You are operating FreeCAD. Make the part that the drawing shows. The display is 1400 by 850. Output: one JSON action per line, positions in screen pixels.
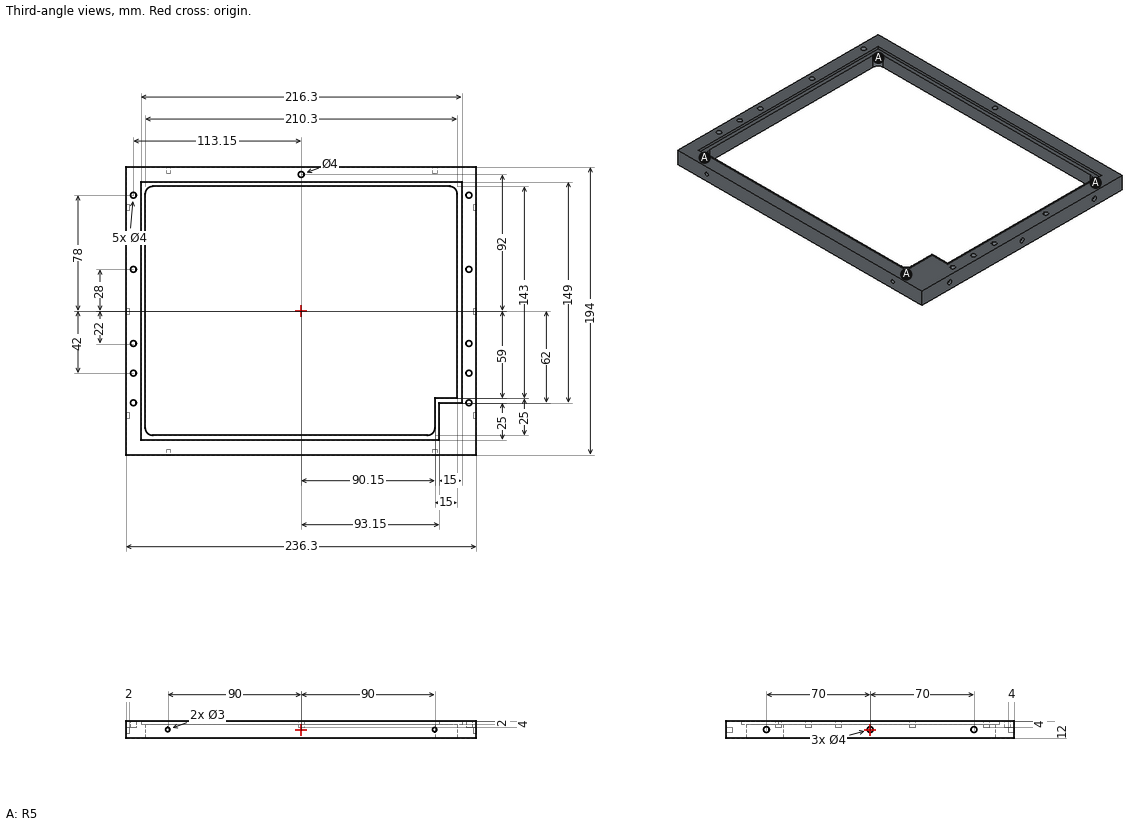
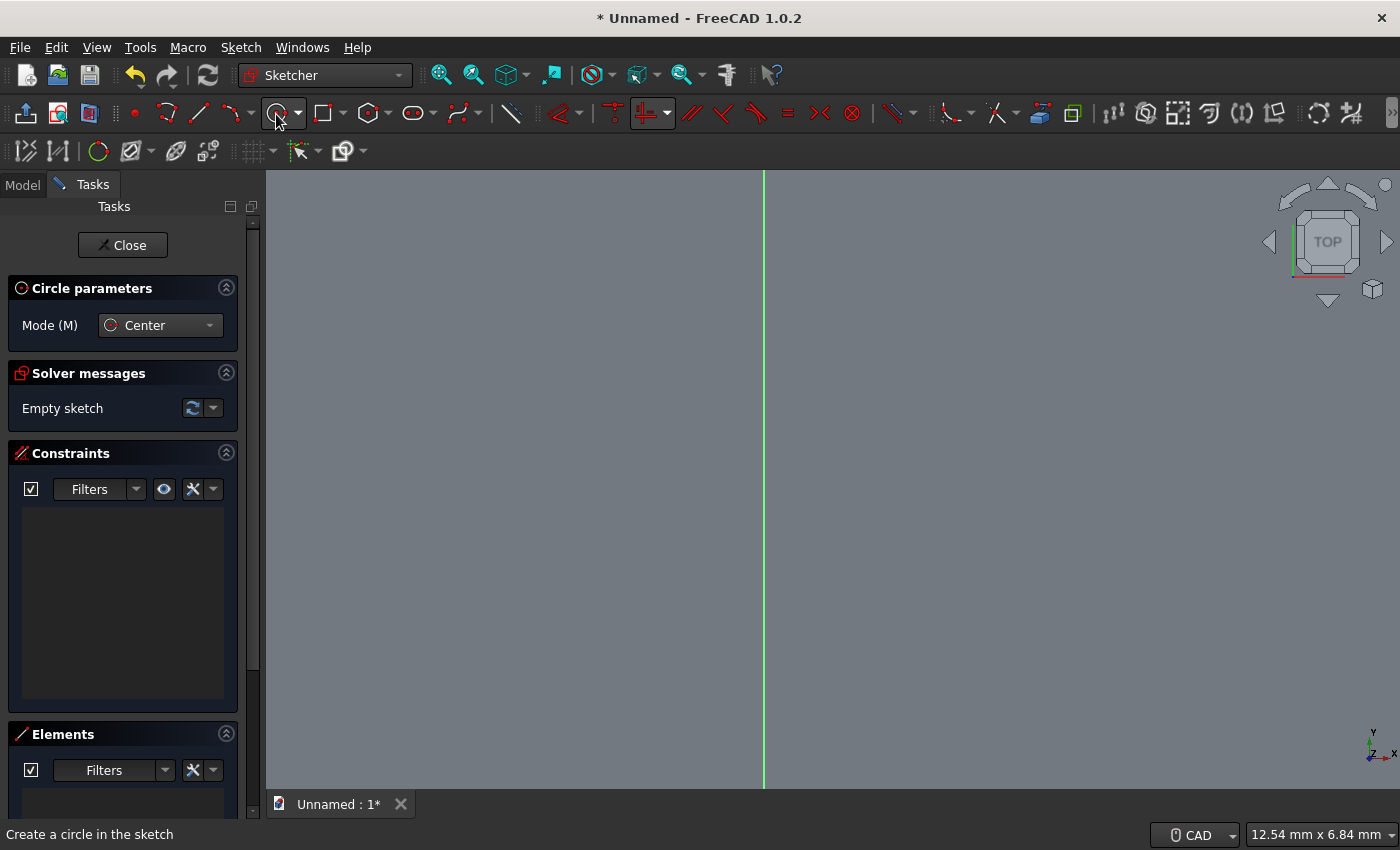
{"action": "left_click", "coordinate": [764, 479]}
{"action": "left_click", "coordinate": [892, 351]}
{"action": "key", "text": "Escape"}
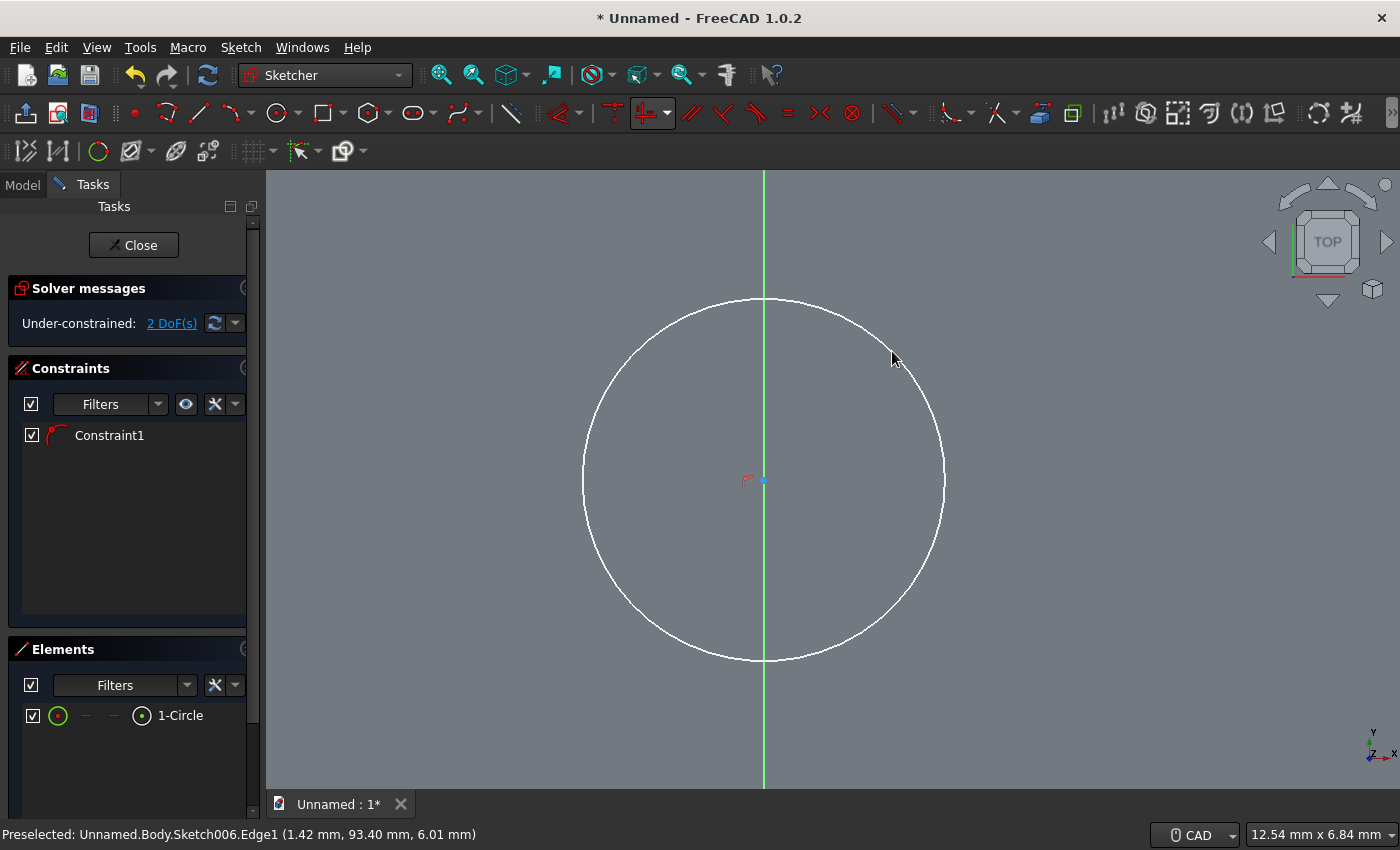
{"action": "left_click", "coordinate": [558, 114]}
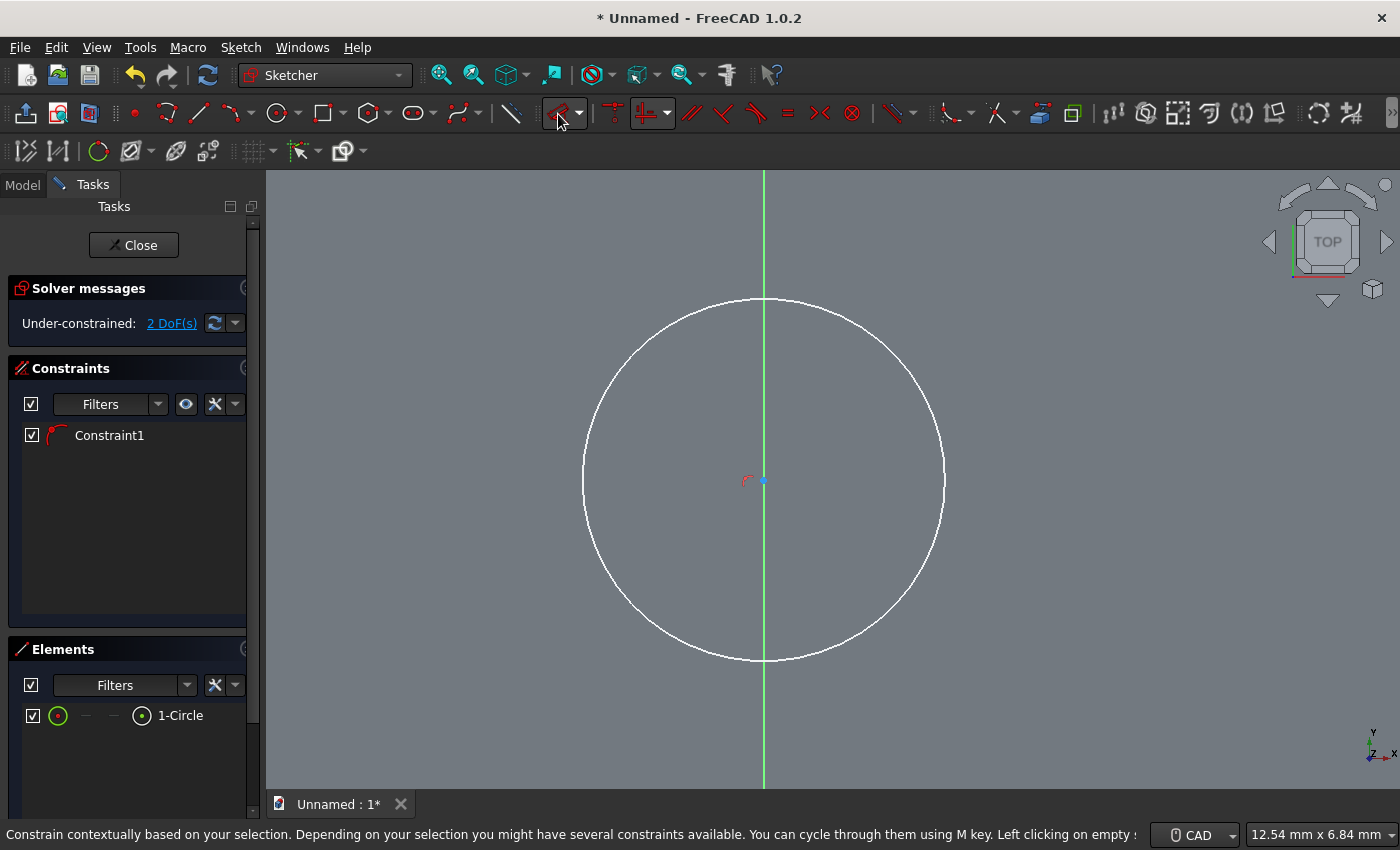
{"action": "left_click", "coordinate": [891, 351]}
{"action": "left_click", "coordinate": [913, 328]}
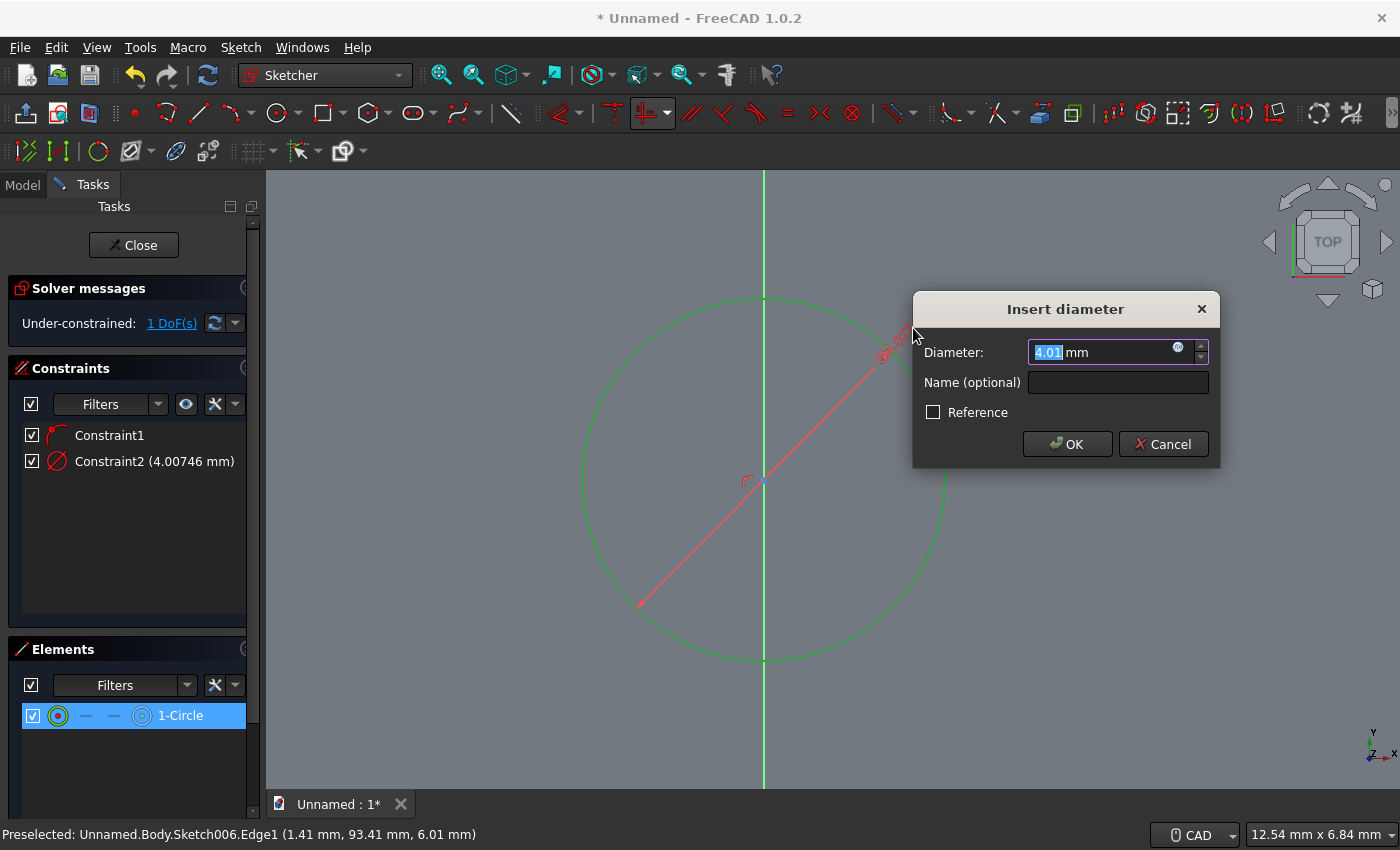
{"action": "type", "text": "4"}
{"action": "key", "text": "Return"}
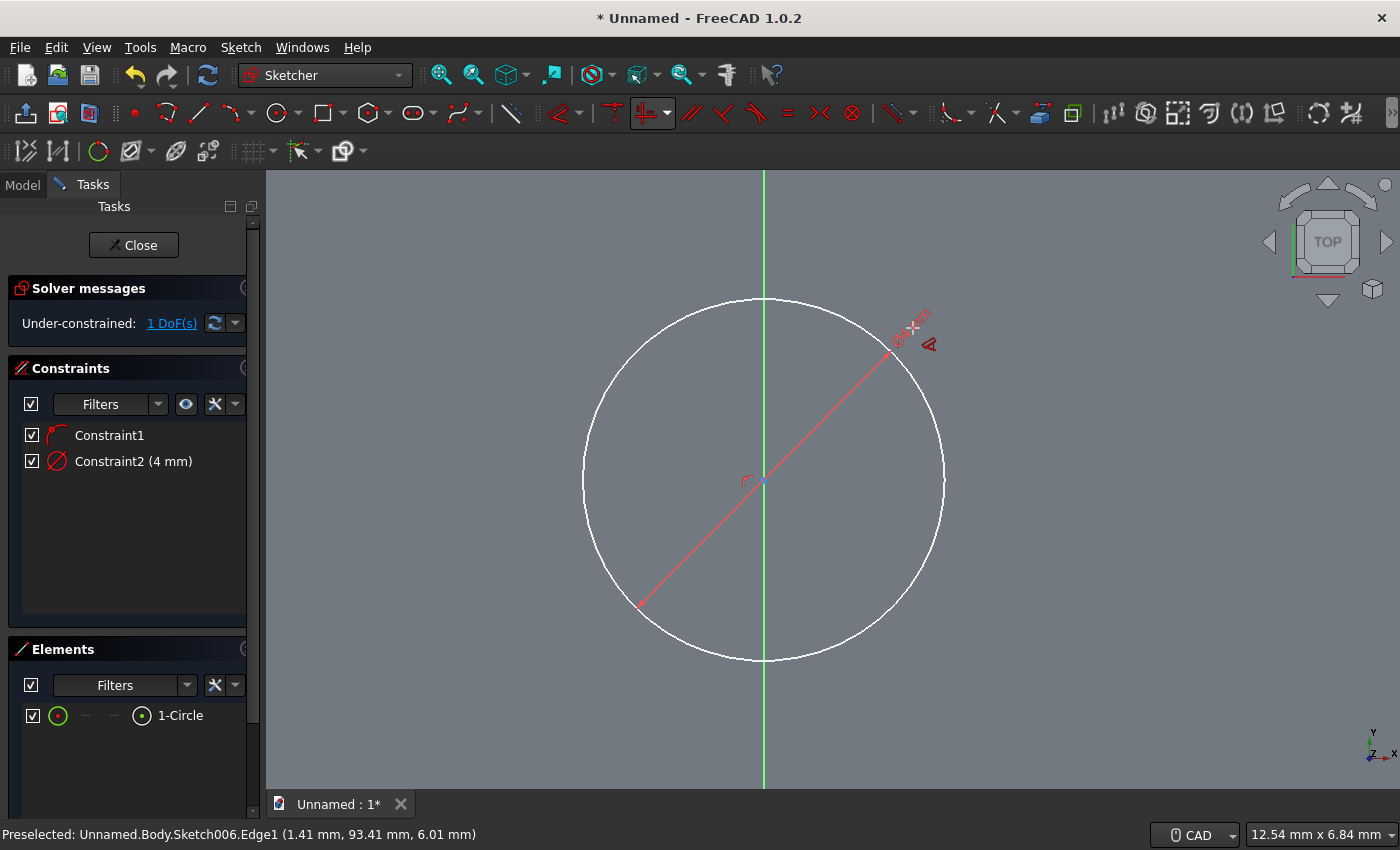
{"action": "left_click", "coordinate": [764, 480]}
{"action": "left_click", "coordinate": [798, 621]}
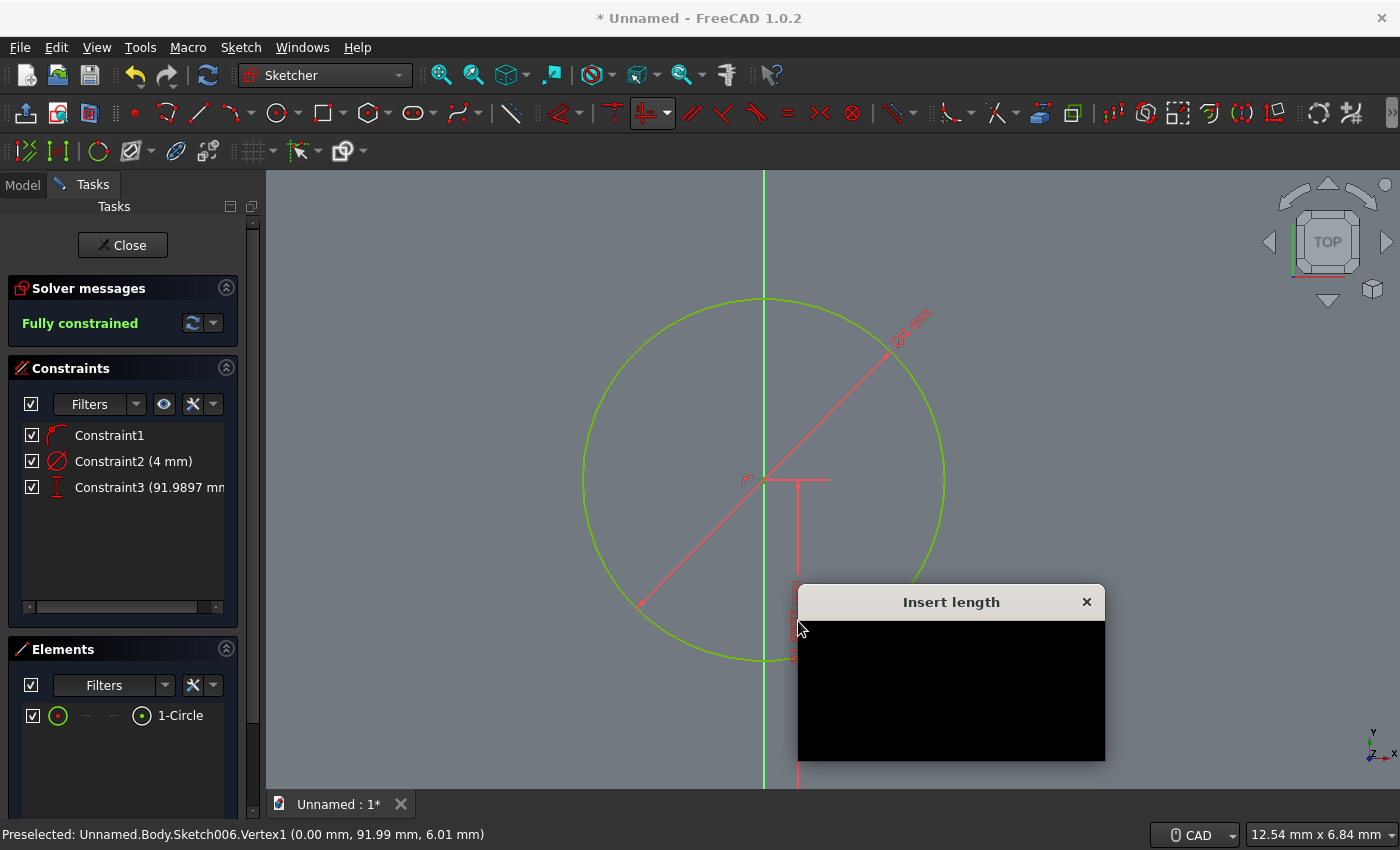
{"action": "type", "text": "92"}
{"action": "key", "text": "Return"}
{"action": "key", "text": "Escape"}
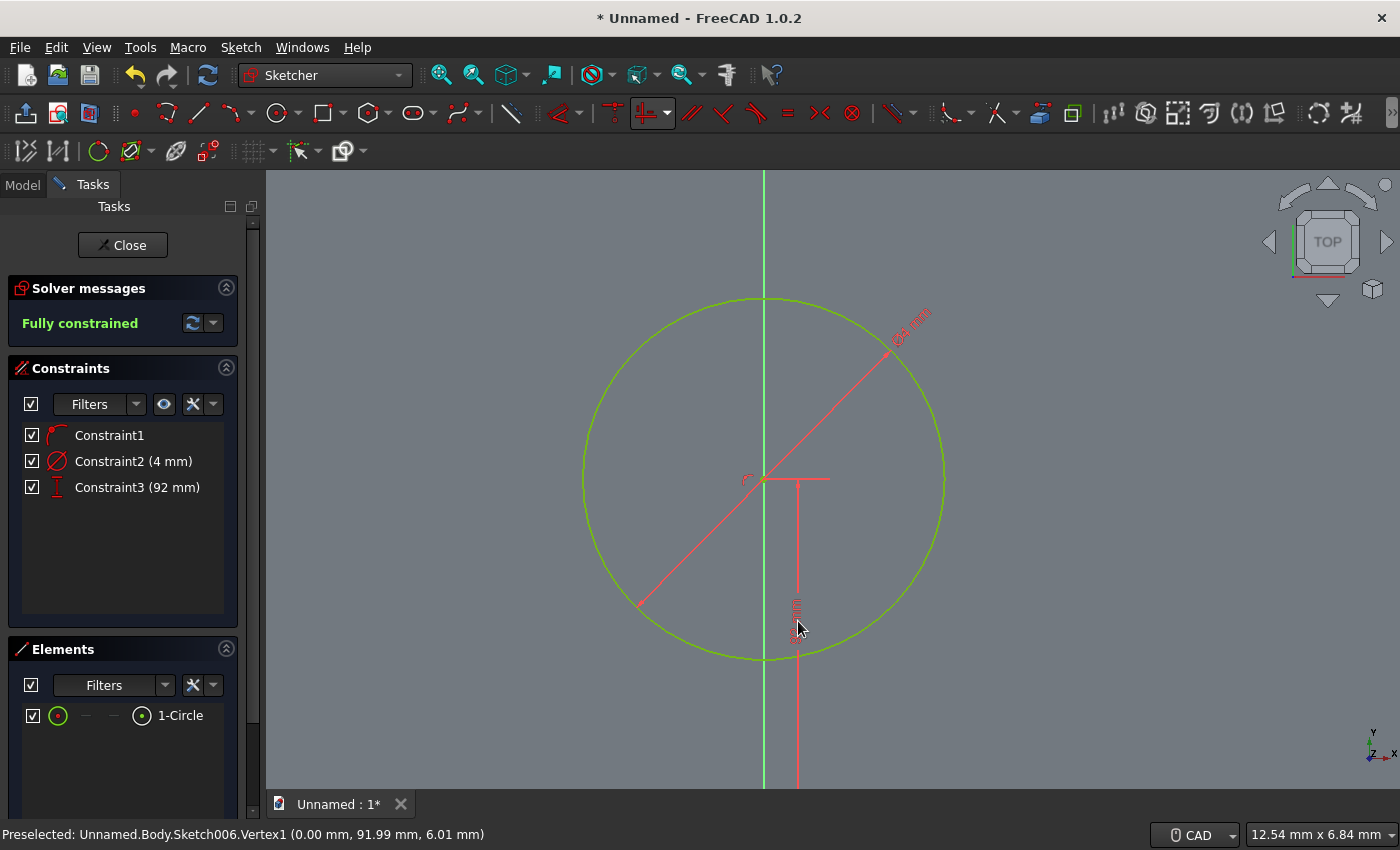
{"action": "left_click", "coordinate": [123, 245]}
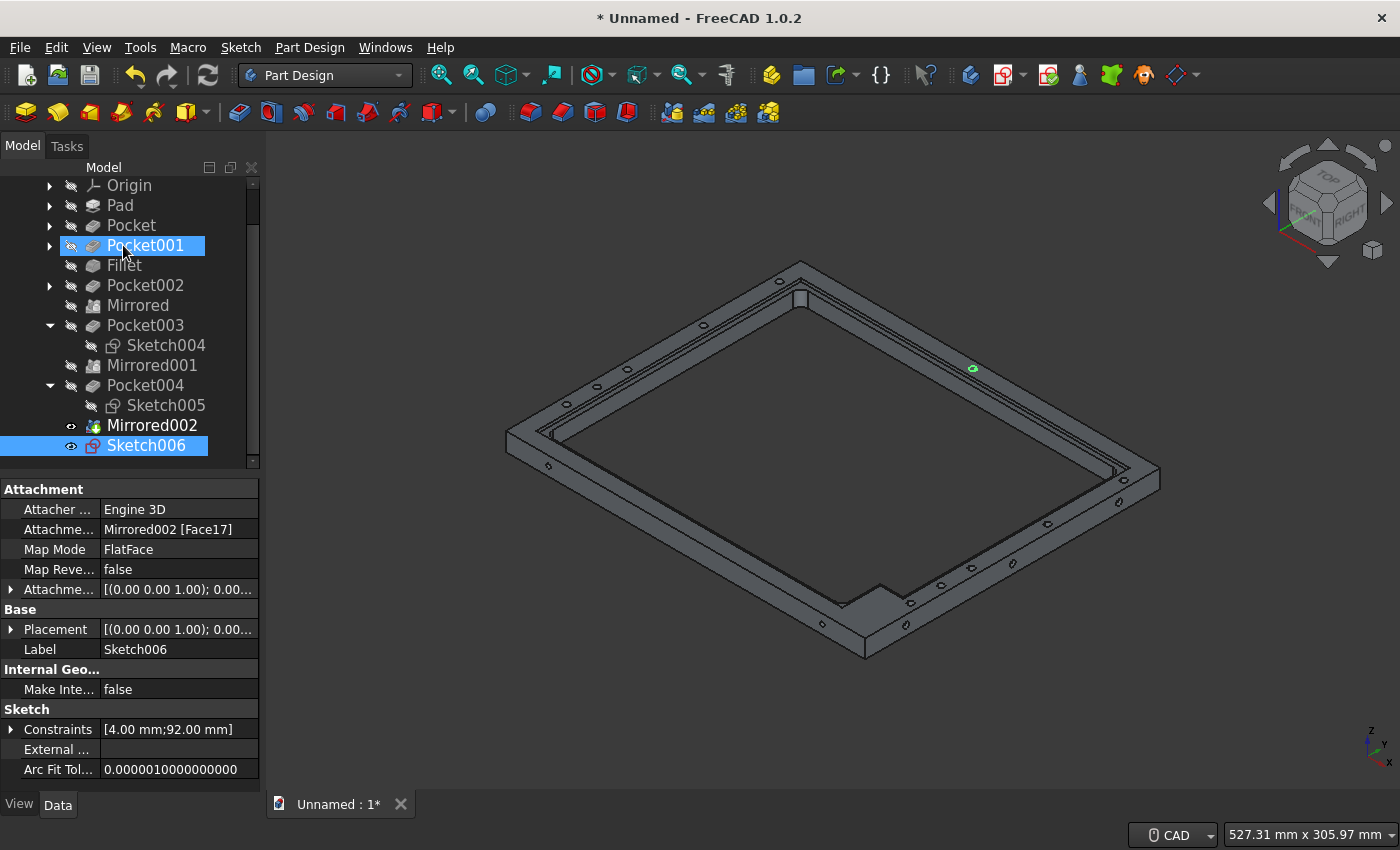
{"action": "left_click", "coordinate": [240, 112]}